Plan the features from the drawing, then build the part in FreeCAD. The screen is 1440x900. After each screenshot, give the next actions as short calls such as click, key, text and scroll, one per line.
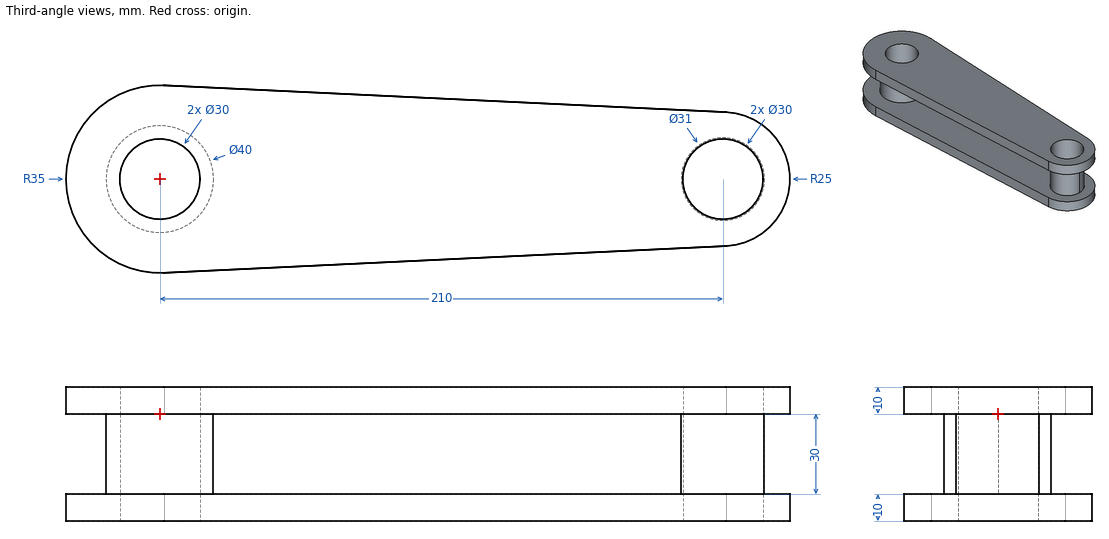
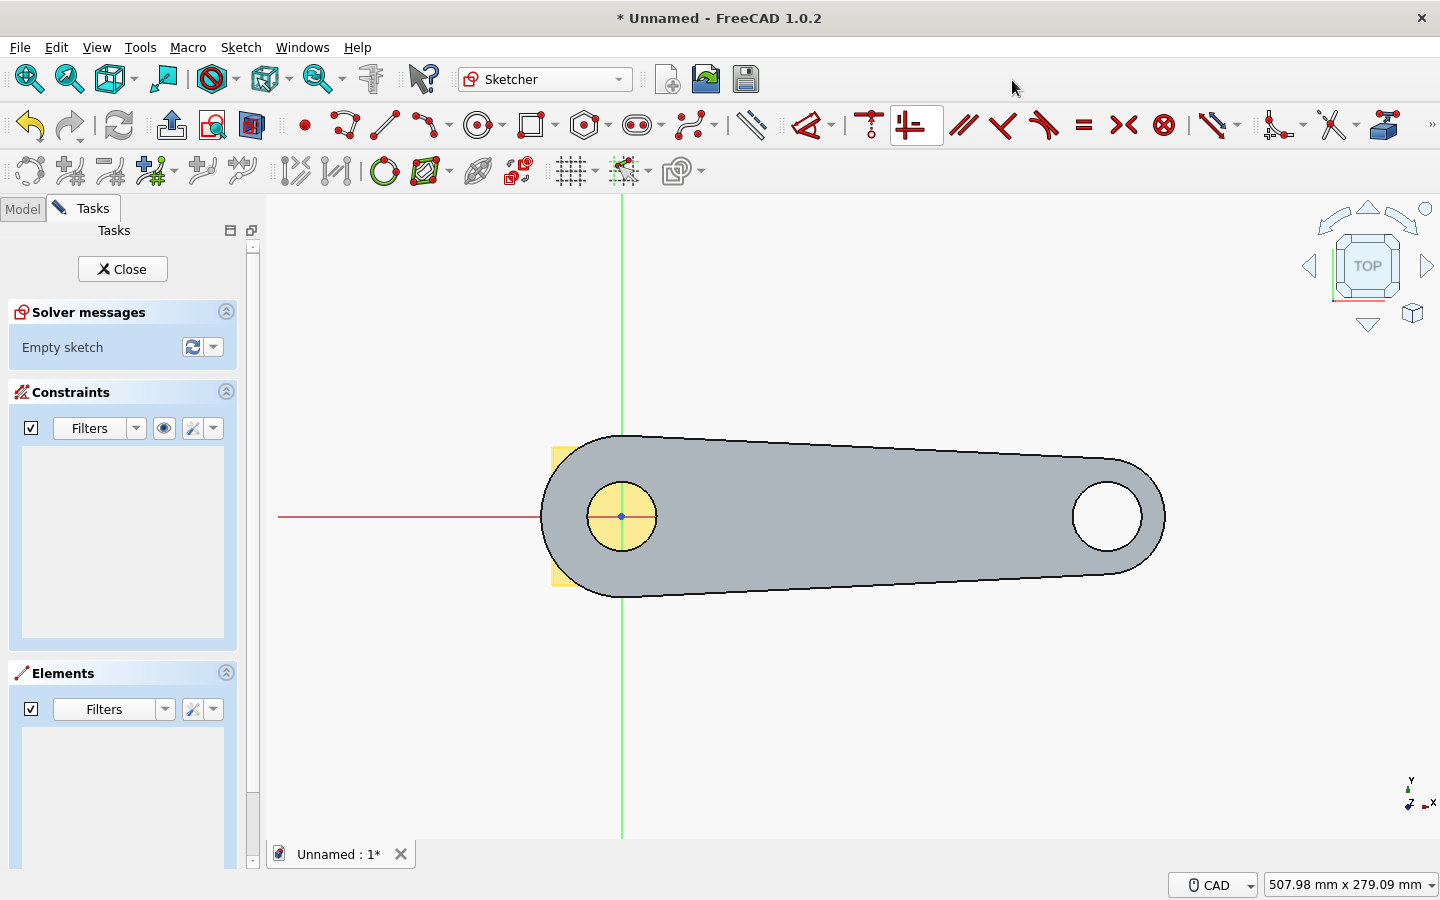
click(386, 126)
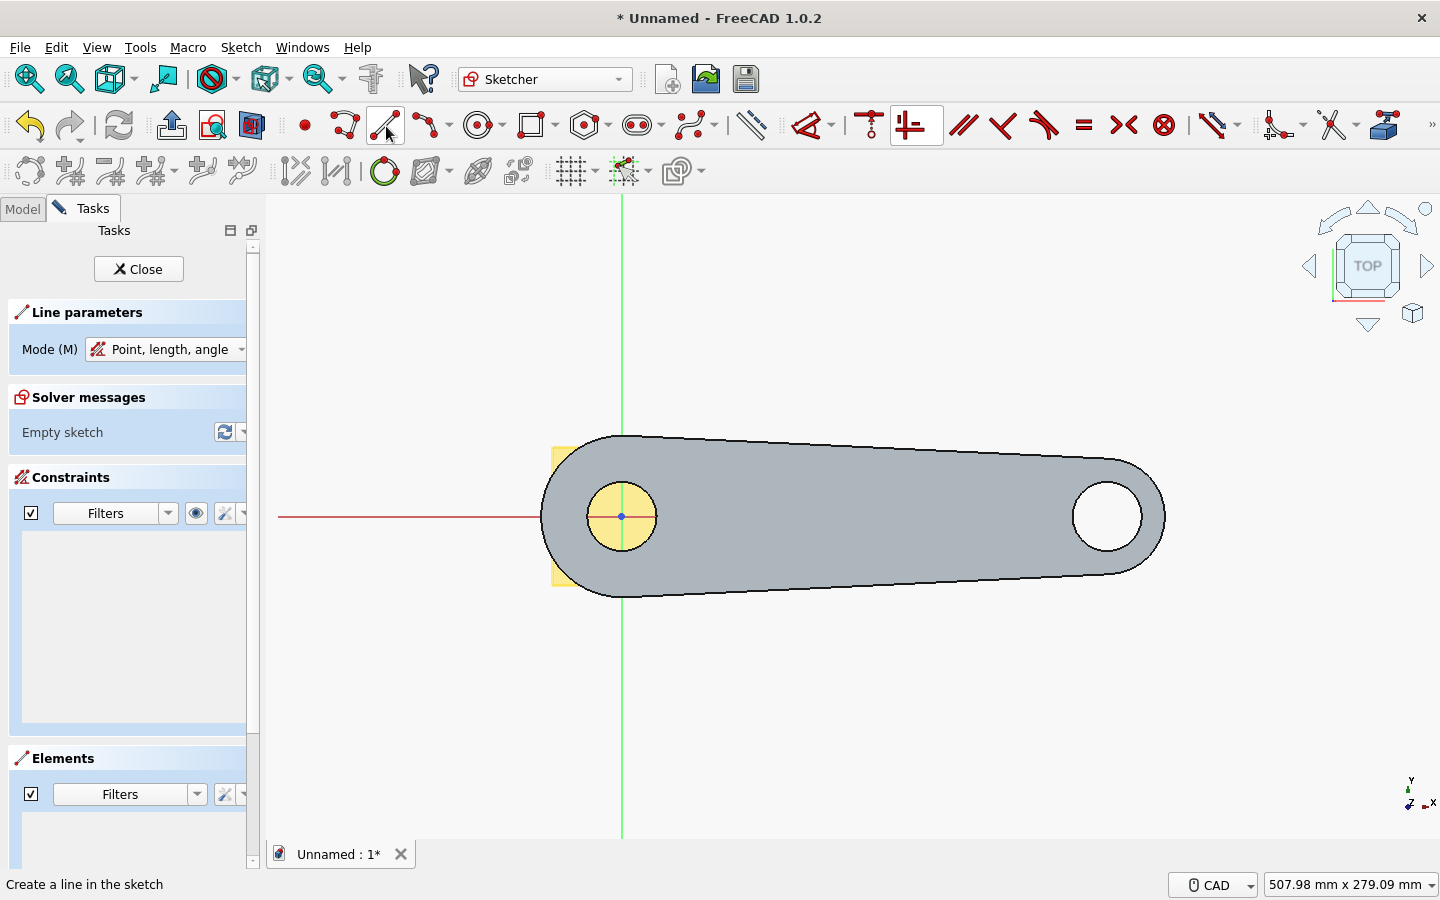
scroll(626, 436, up, 8)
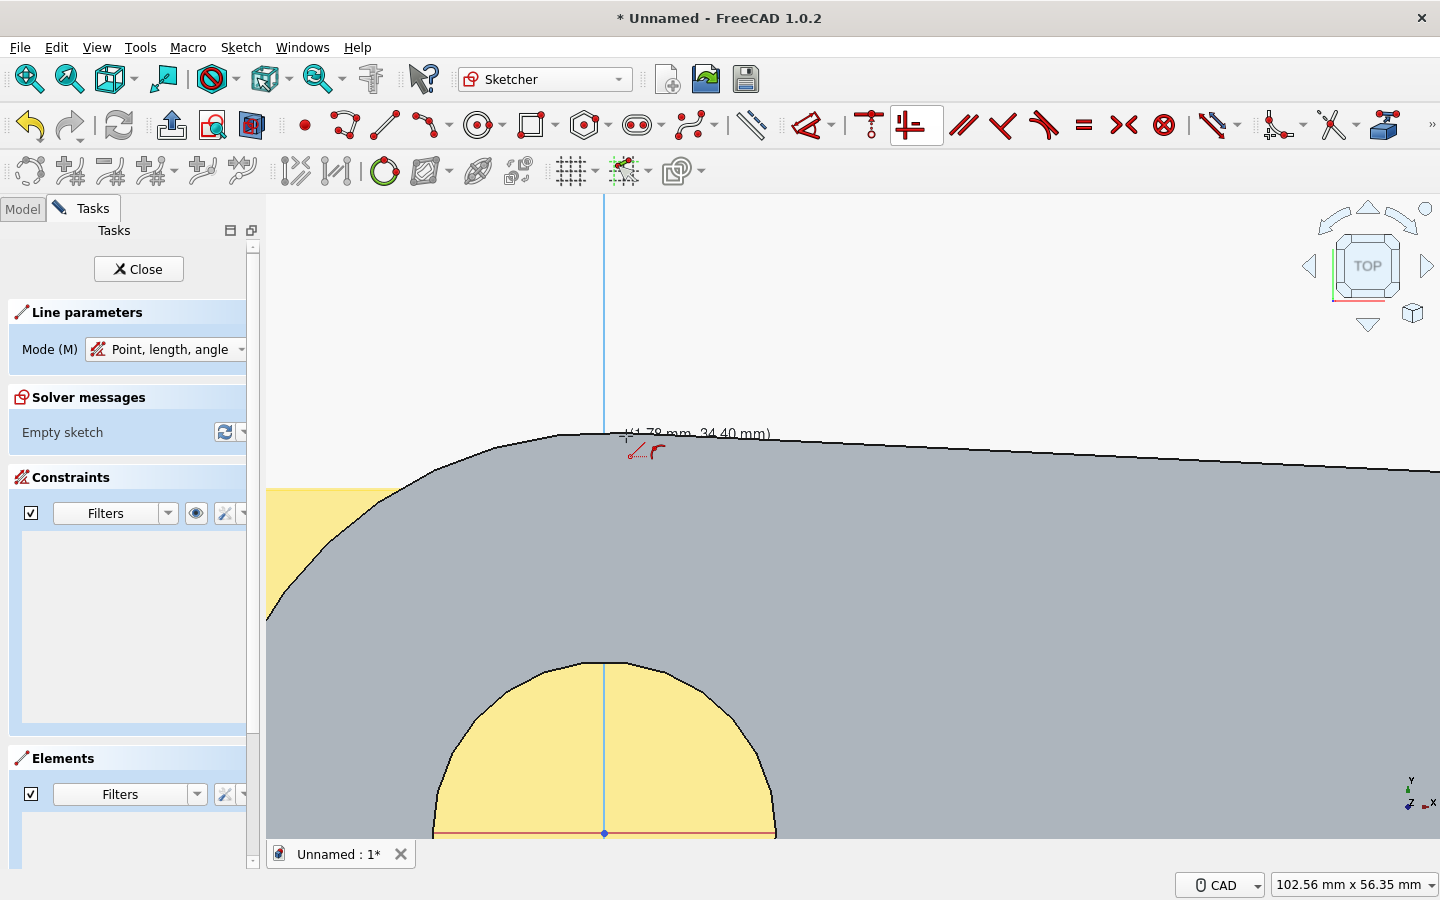
click(623, 433)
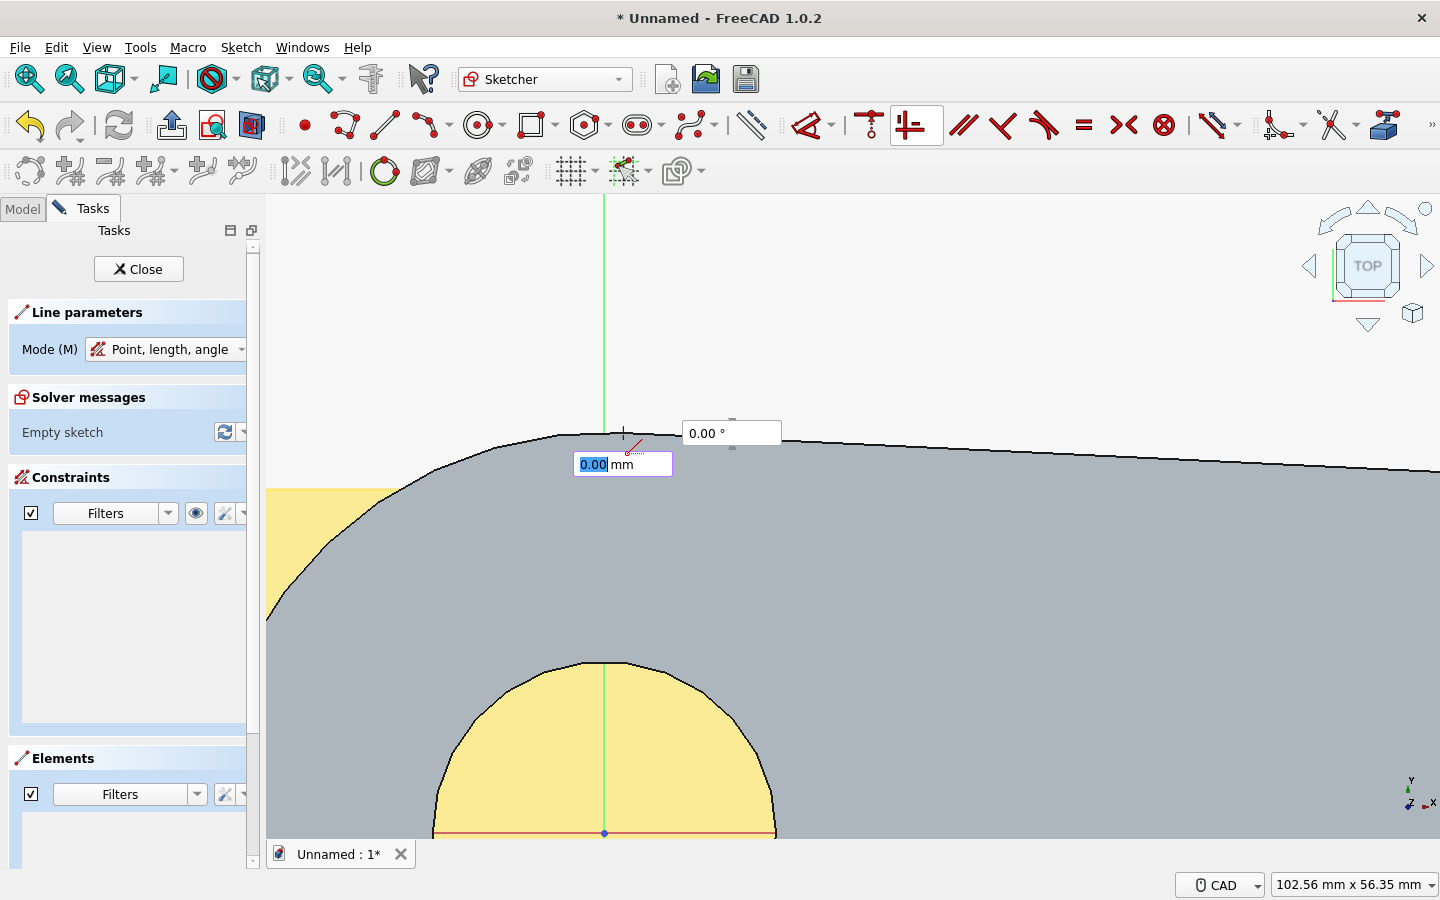
scroll(469, 413, down, 7)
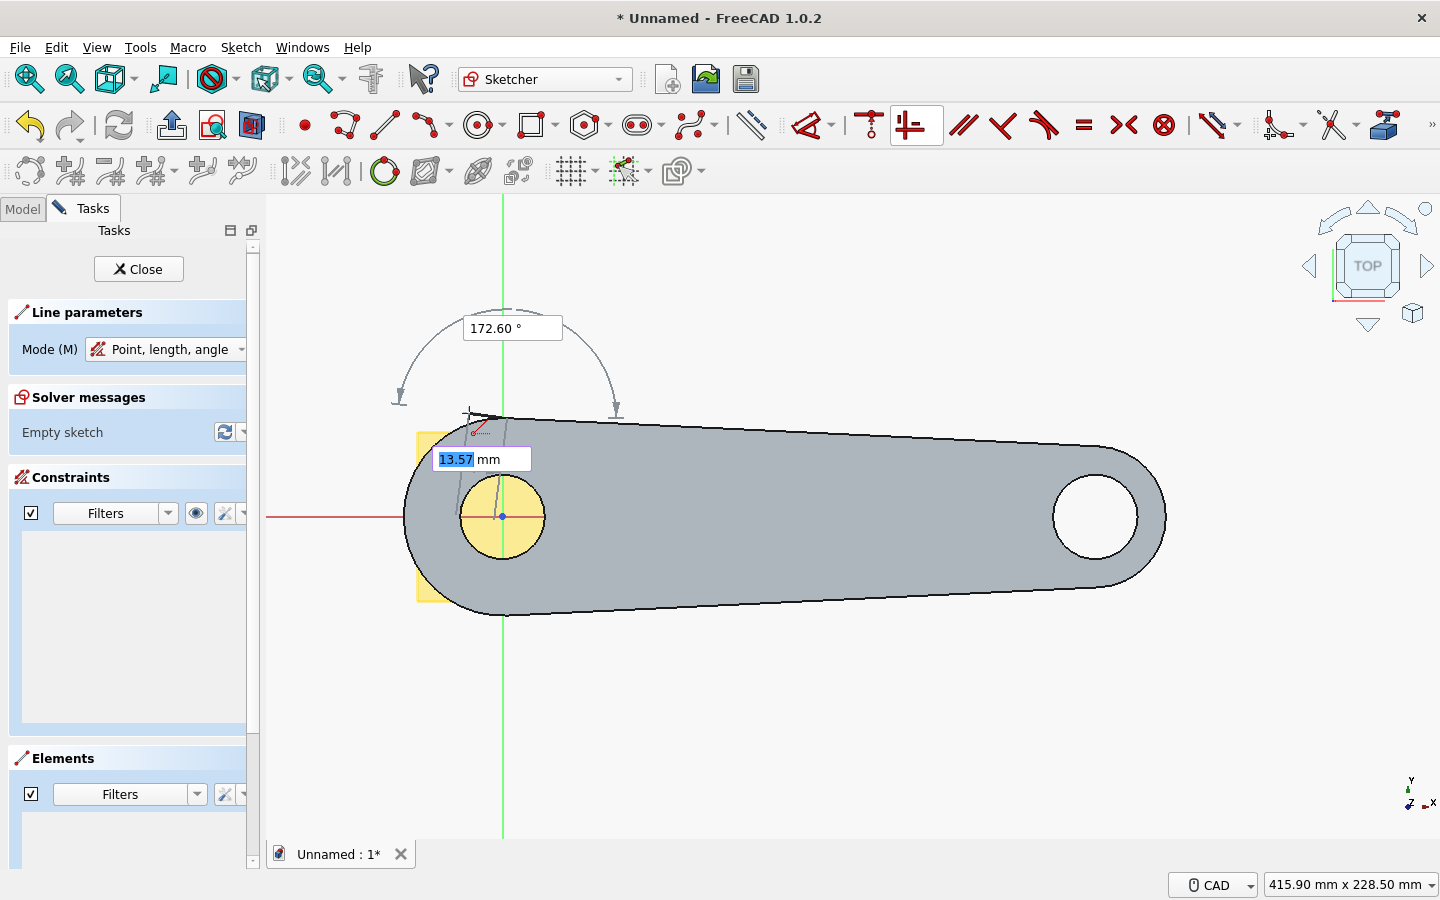
click(1099, 446)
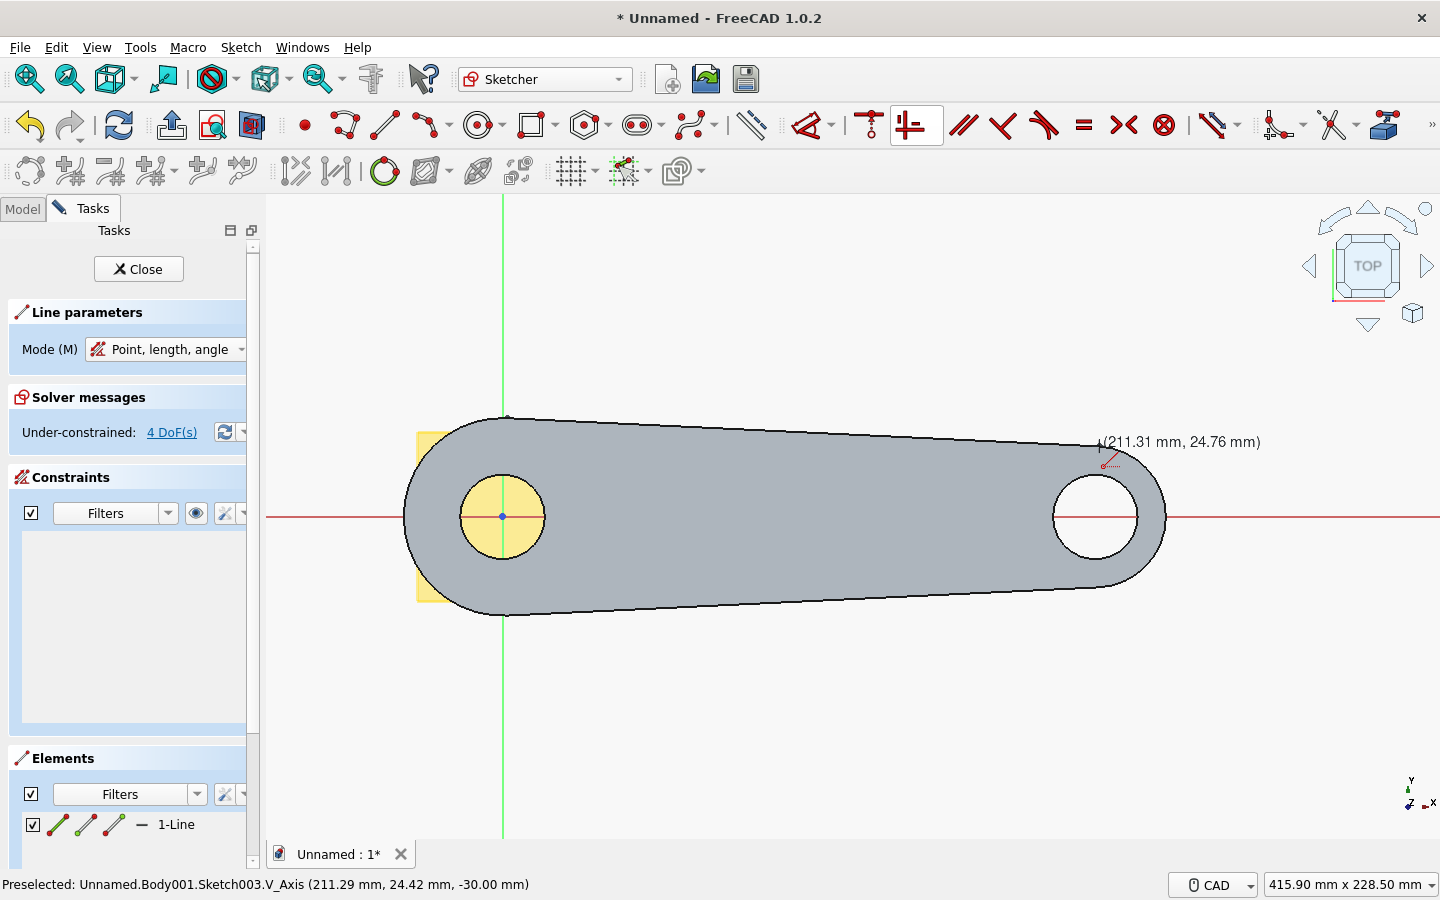
click(1099, 587)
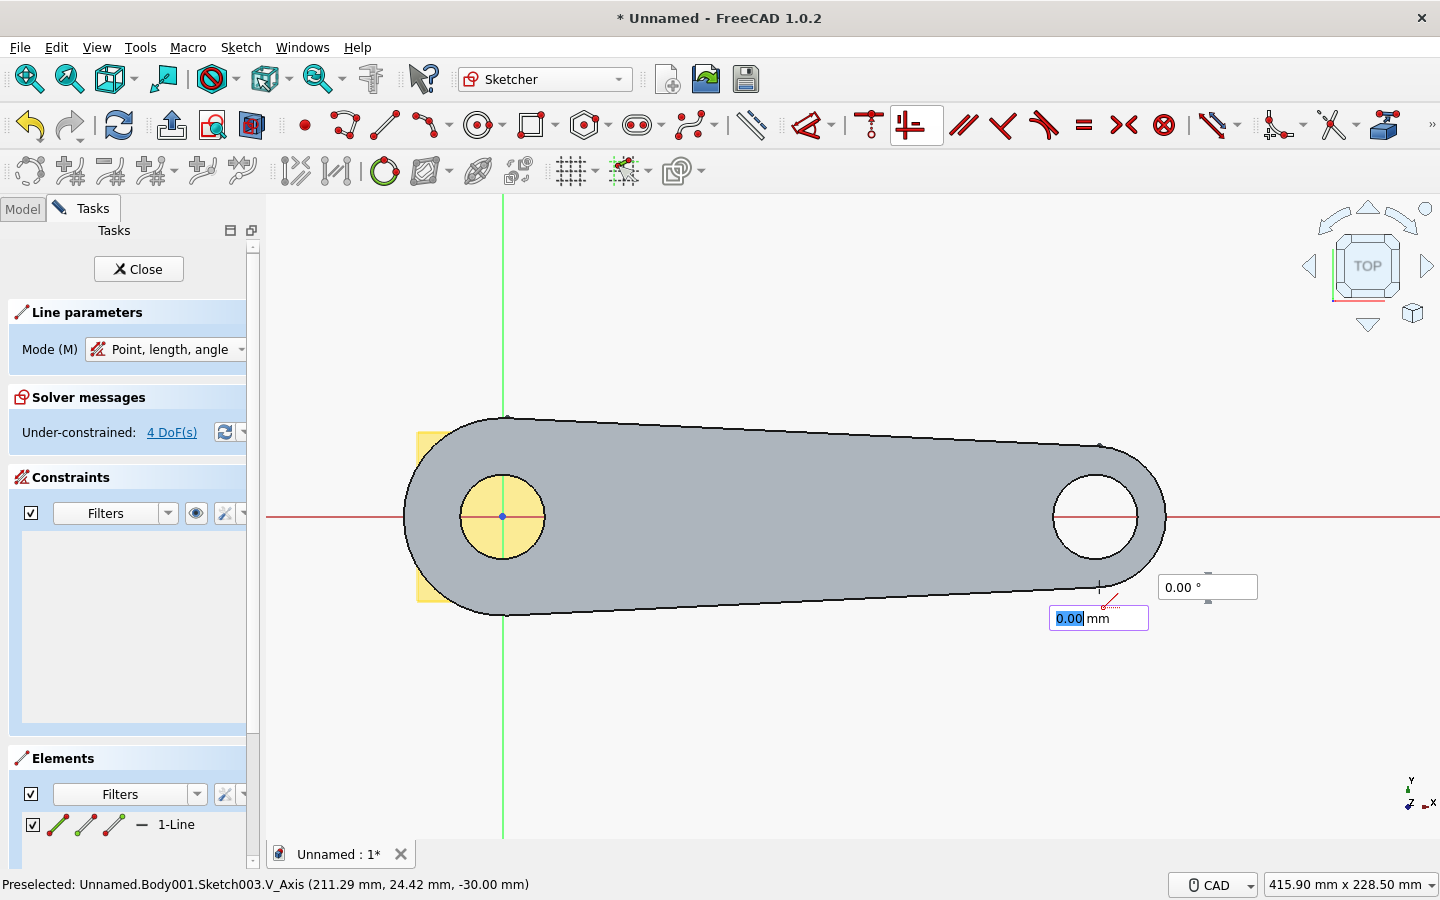
scroll(507, 616, up, 7)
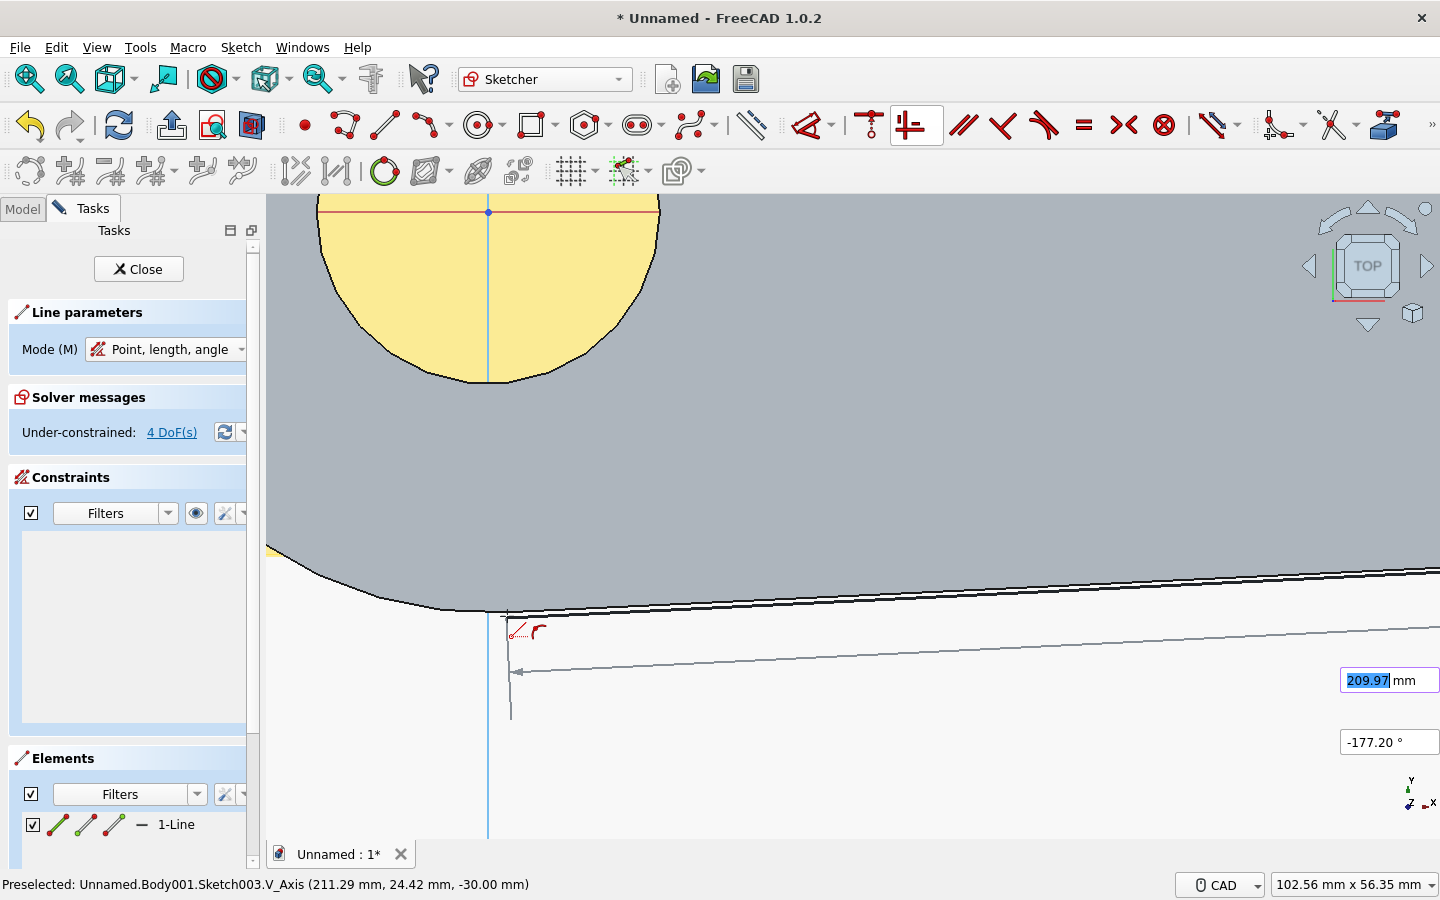
click(507, 612)